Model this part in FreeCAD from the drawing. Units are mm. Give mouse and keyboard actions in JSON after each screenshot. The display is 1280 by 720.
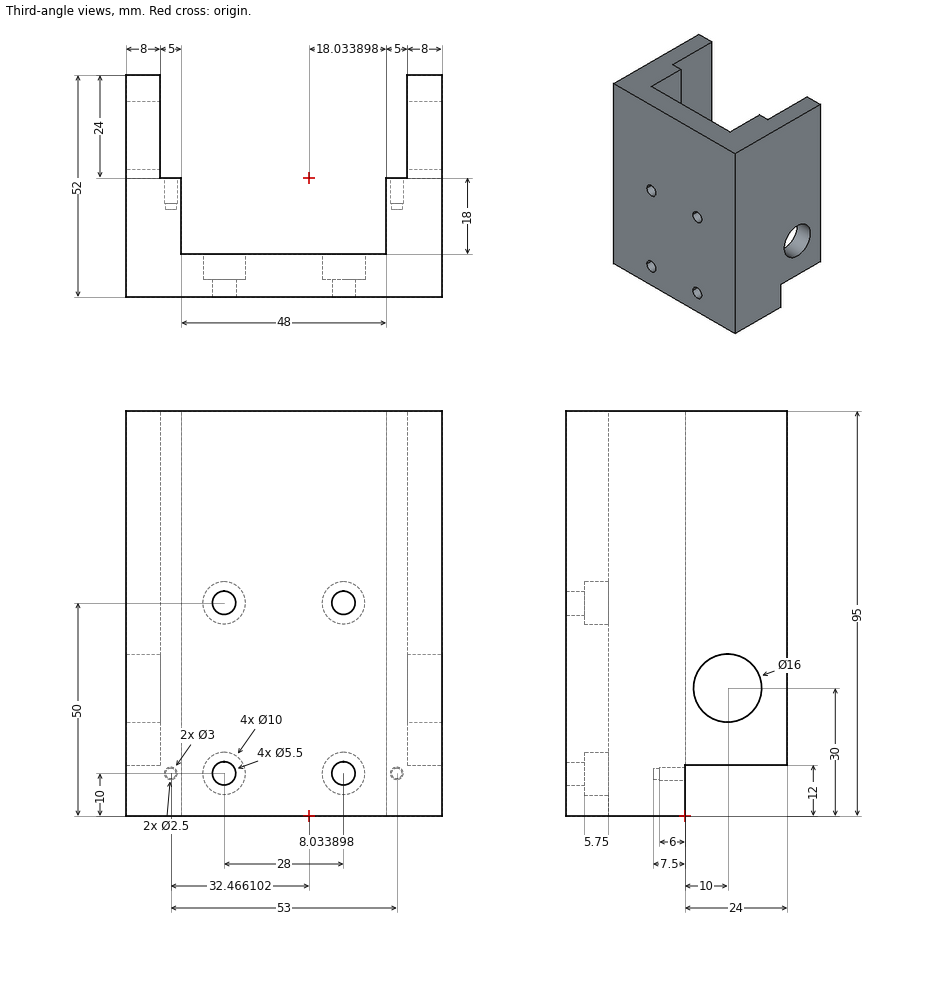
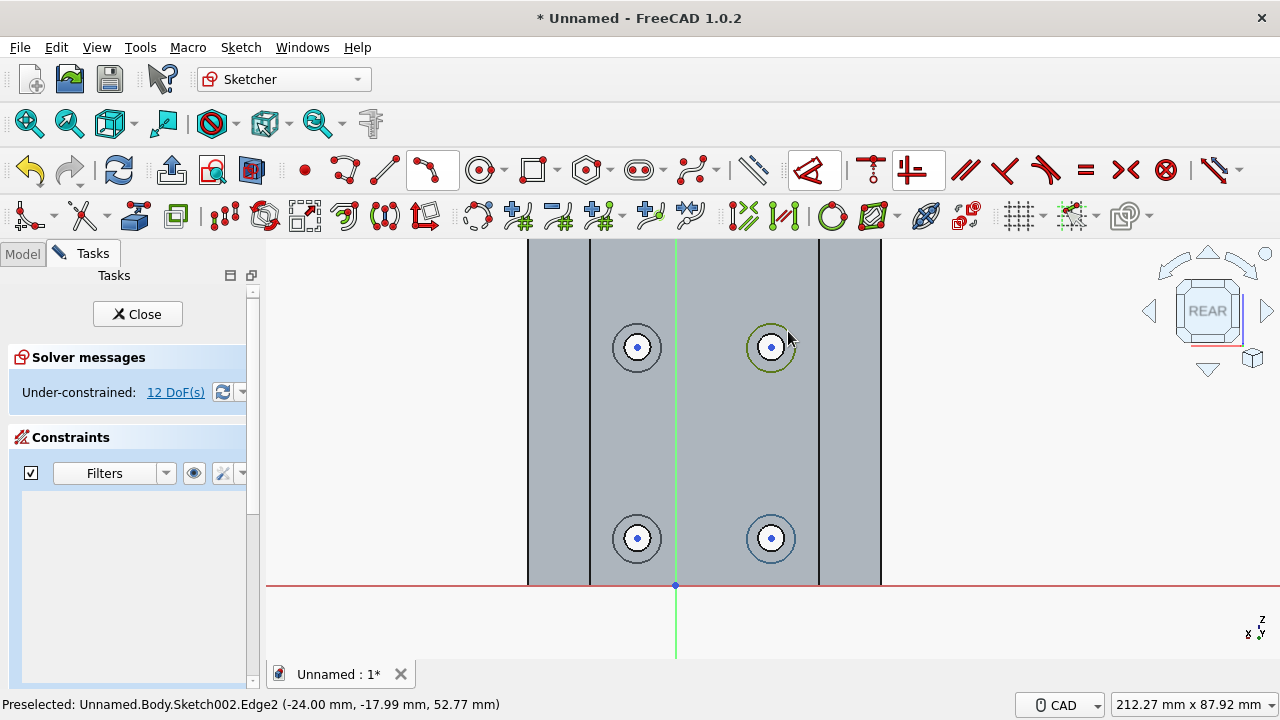
{"action": "left_click", "coordinate": [654, 522]}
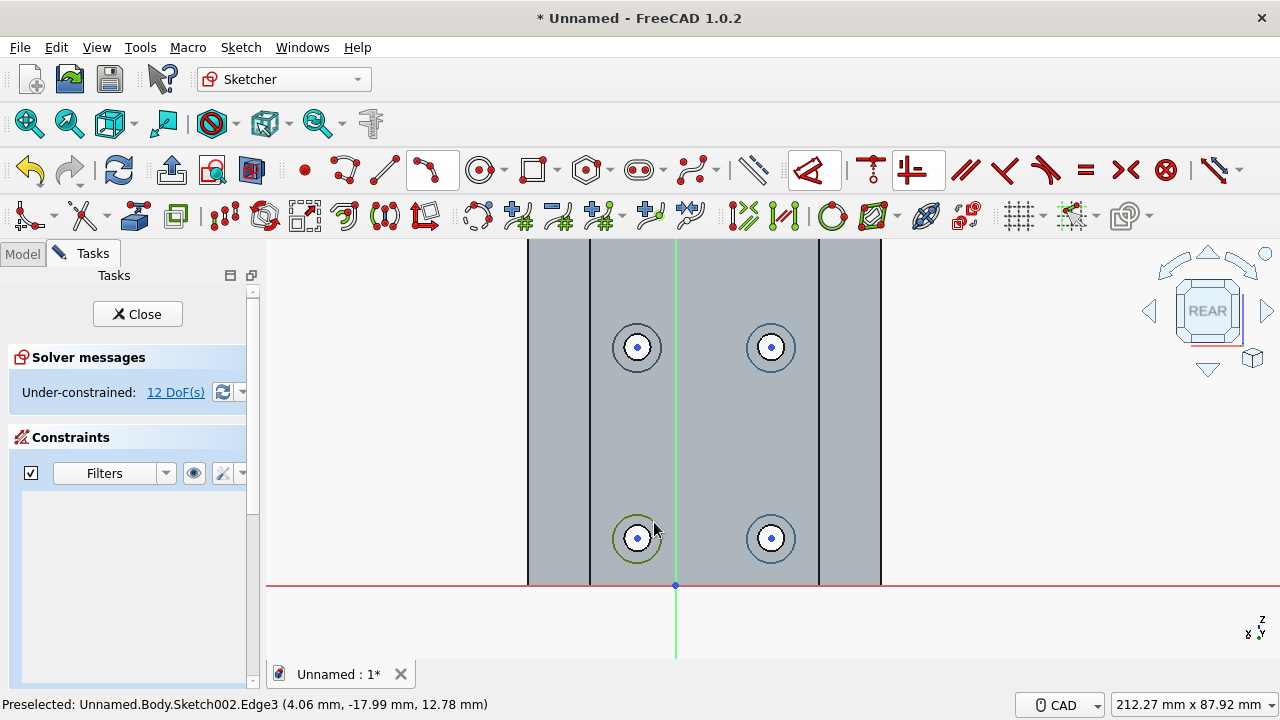
{"action": "left_click", "coordinate": [654, 331]}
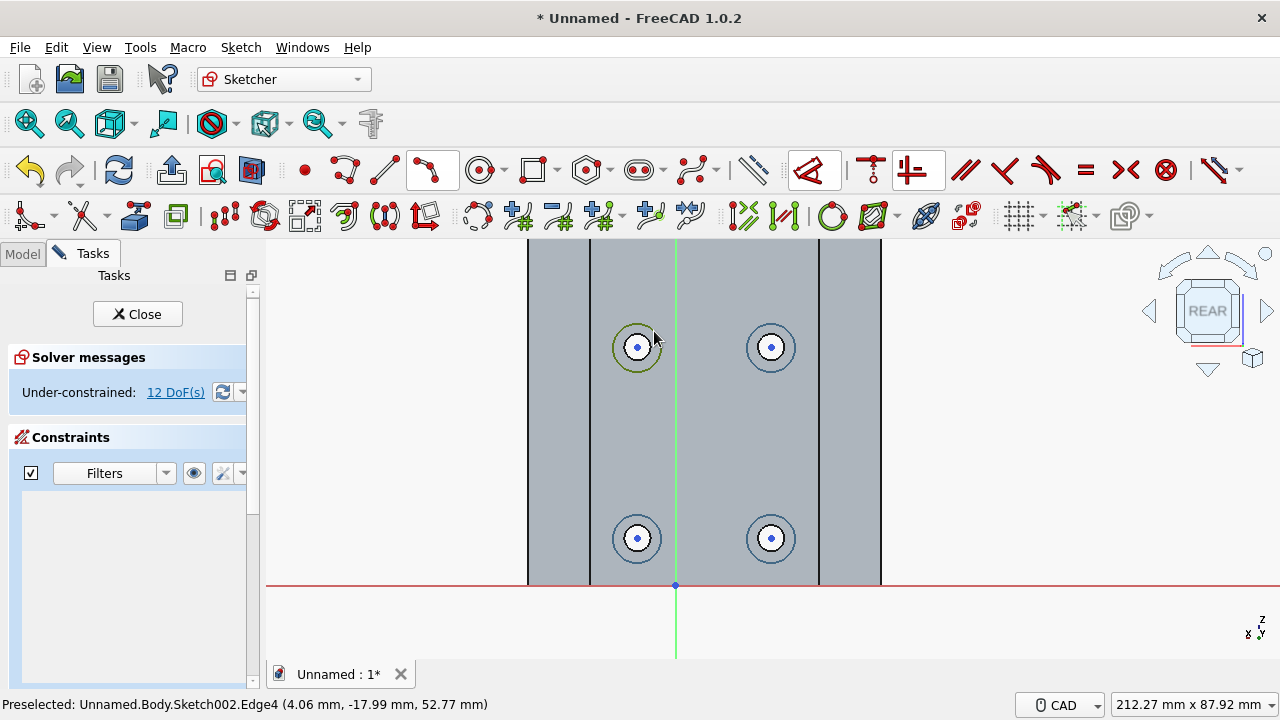
{"action": "key", "text": "e"}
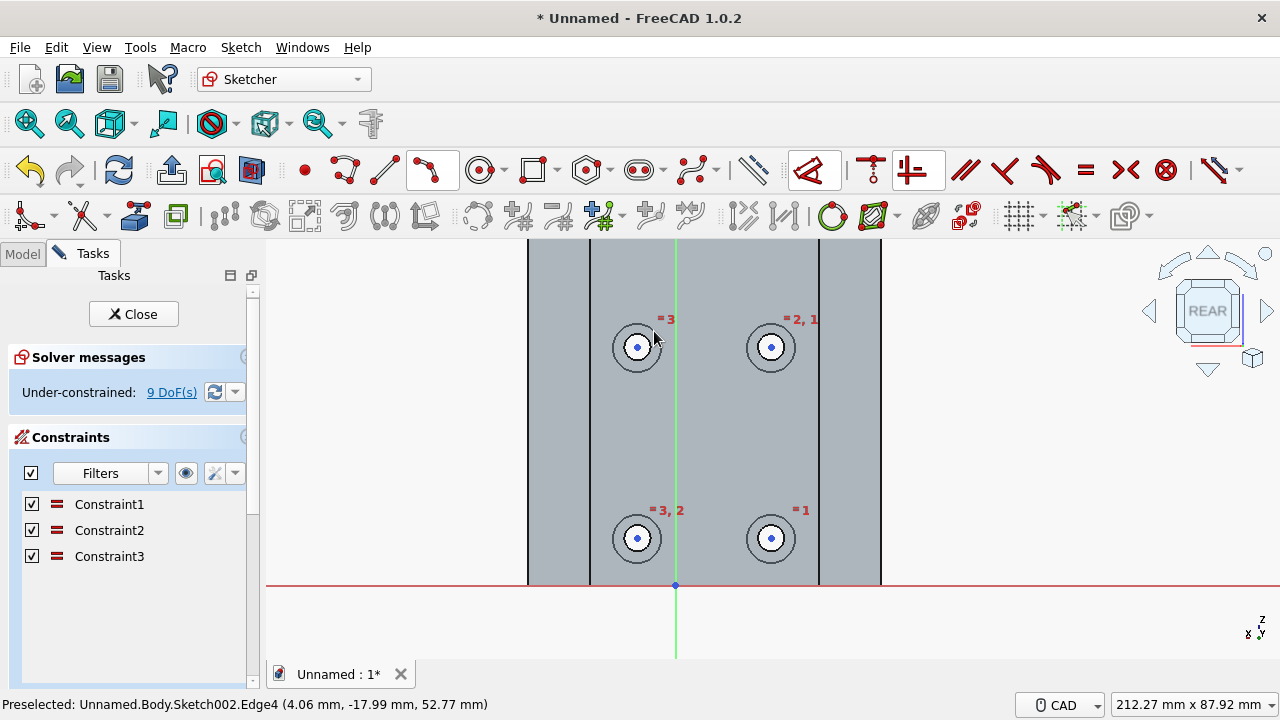
{"action": "left_click", "coordinate": [771, 539]}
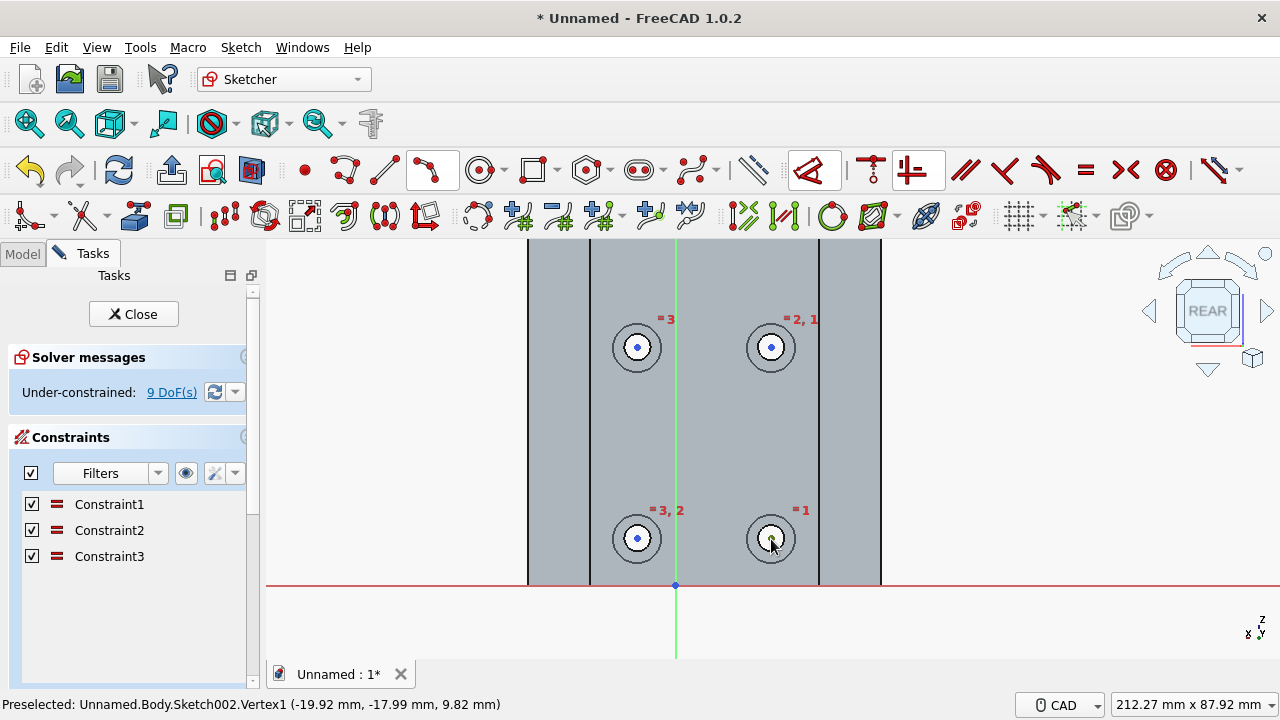
{"action": "left_click", "coordinate": [771, 348]}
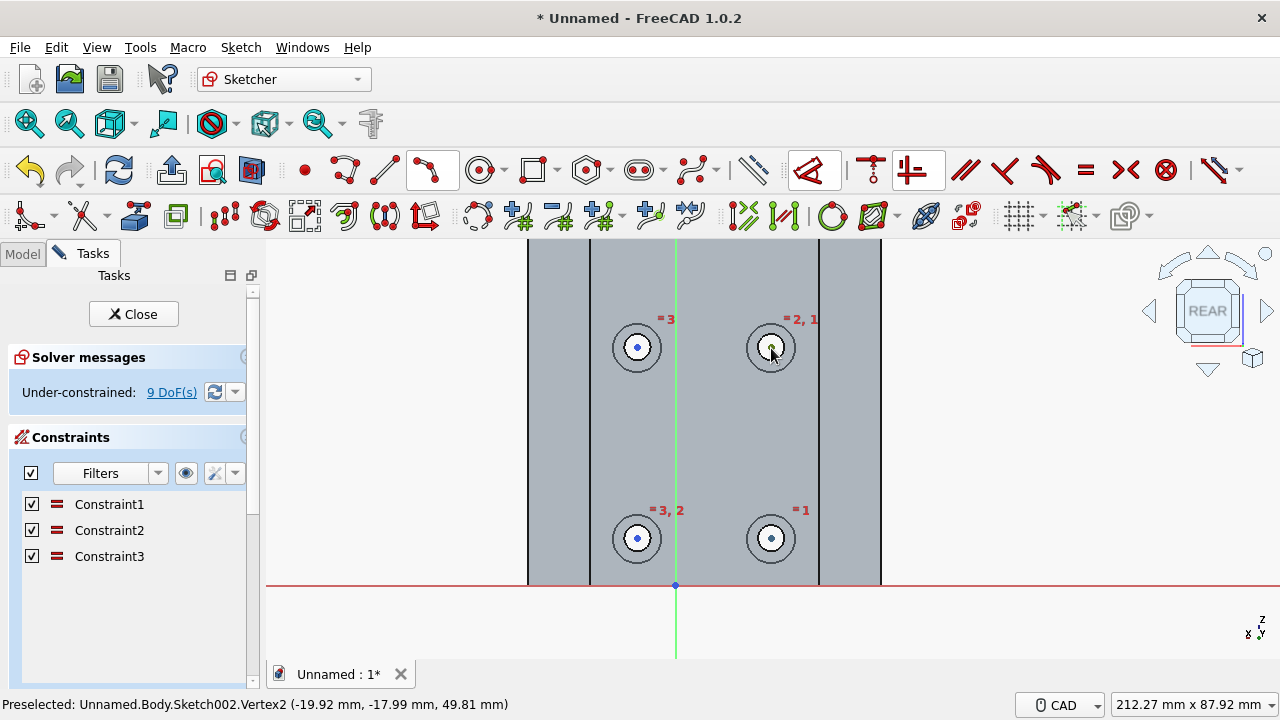
{"action": "key", "text": "v"}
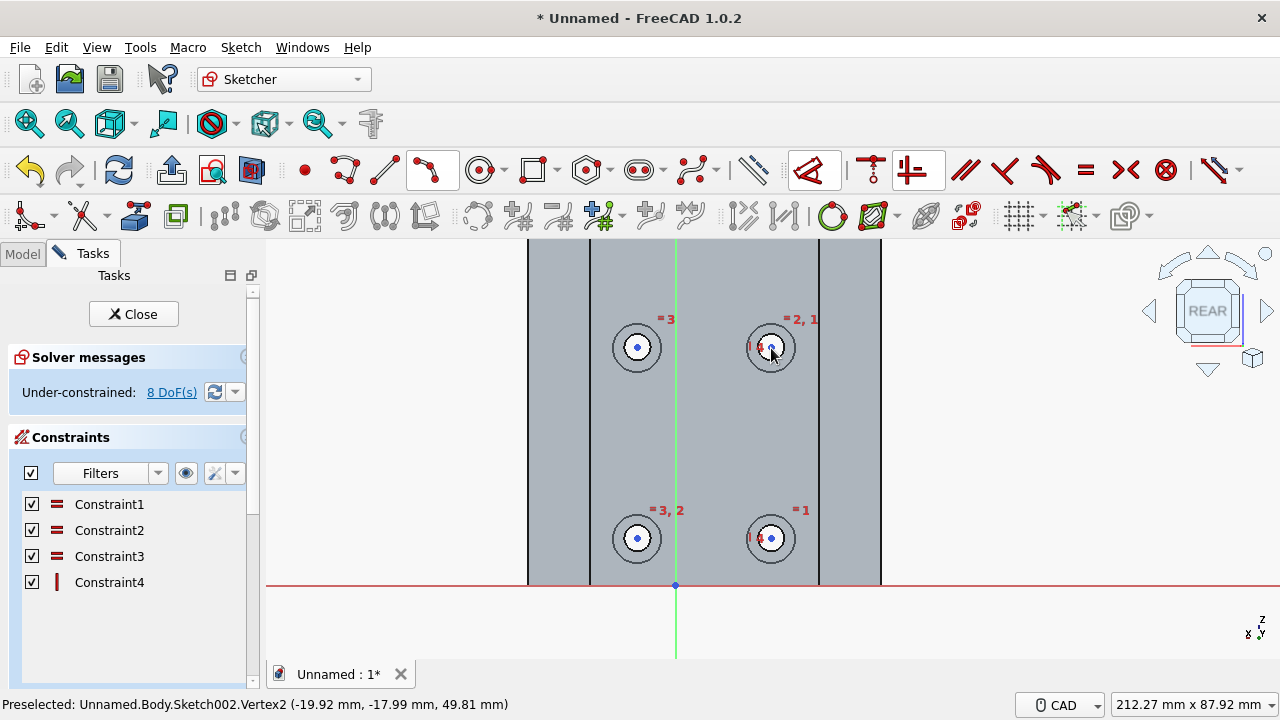
{"action": "left_click", "coordinate": [771, 539]}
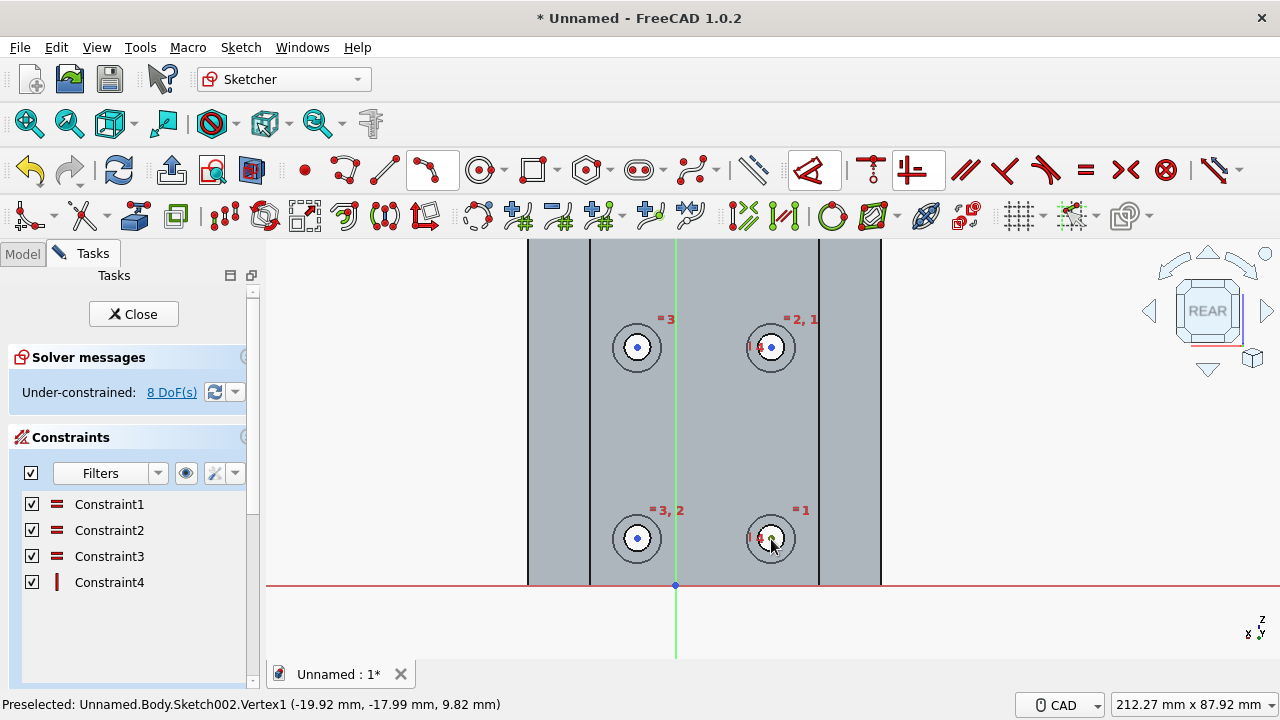
{"action": "left_click", "coordinate": [637, 539]}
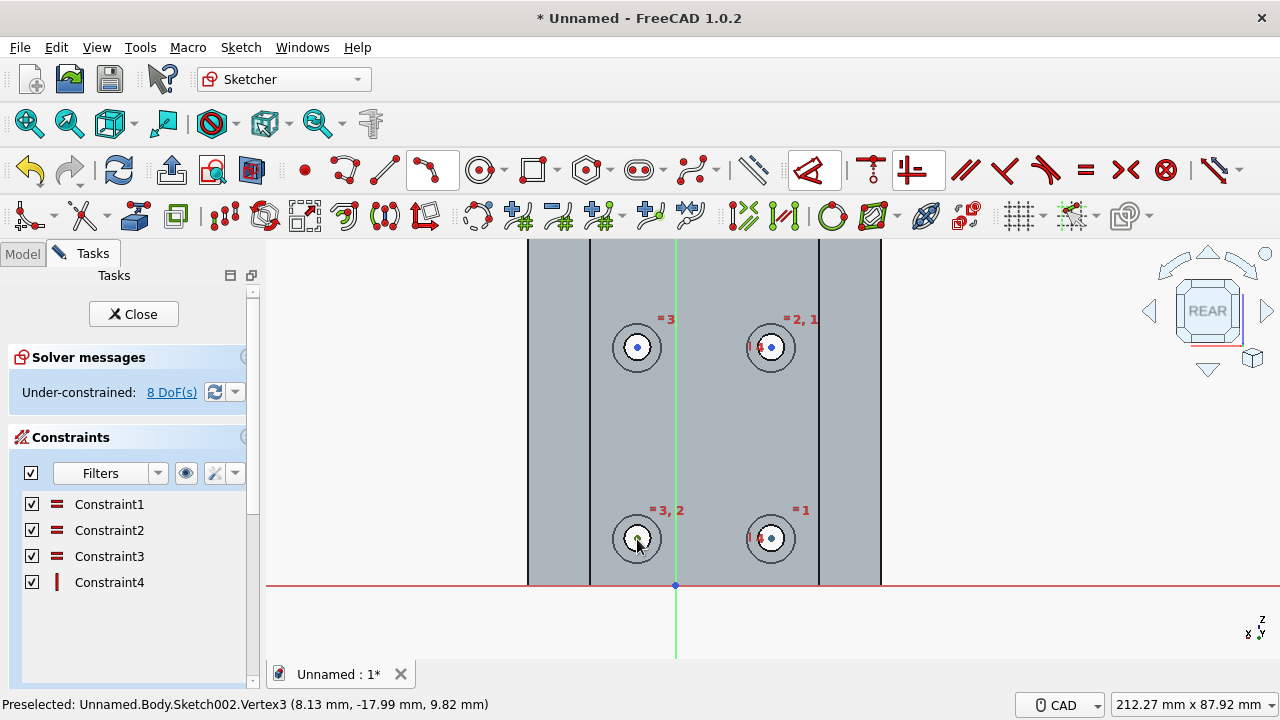
{"action": "left_click", "coordinate": [940, 170]}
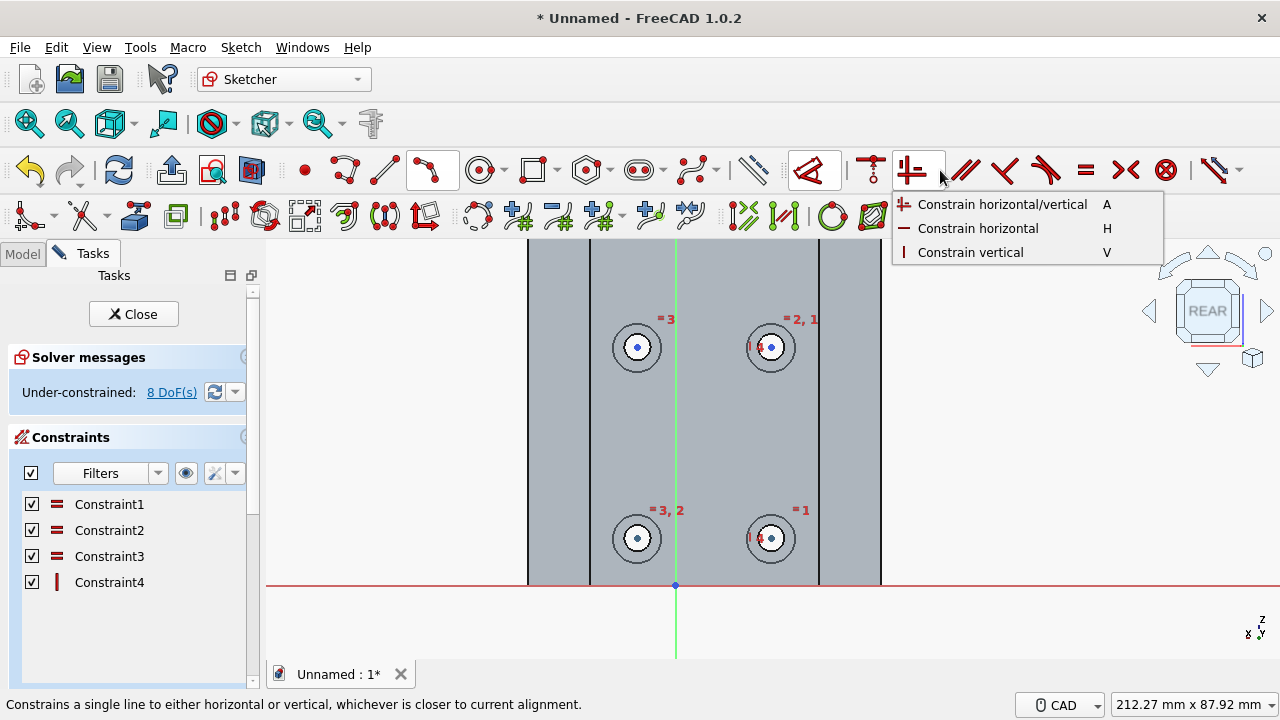
{"action": "left_click", "coordinate": [1028, 228]}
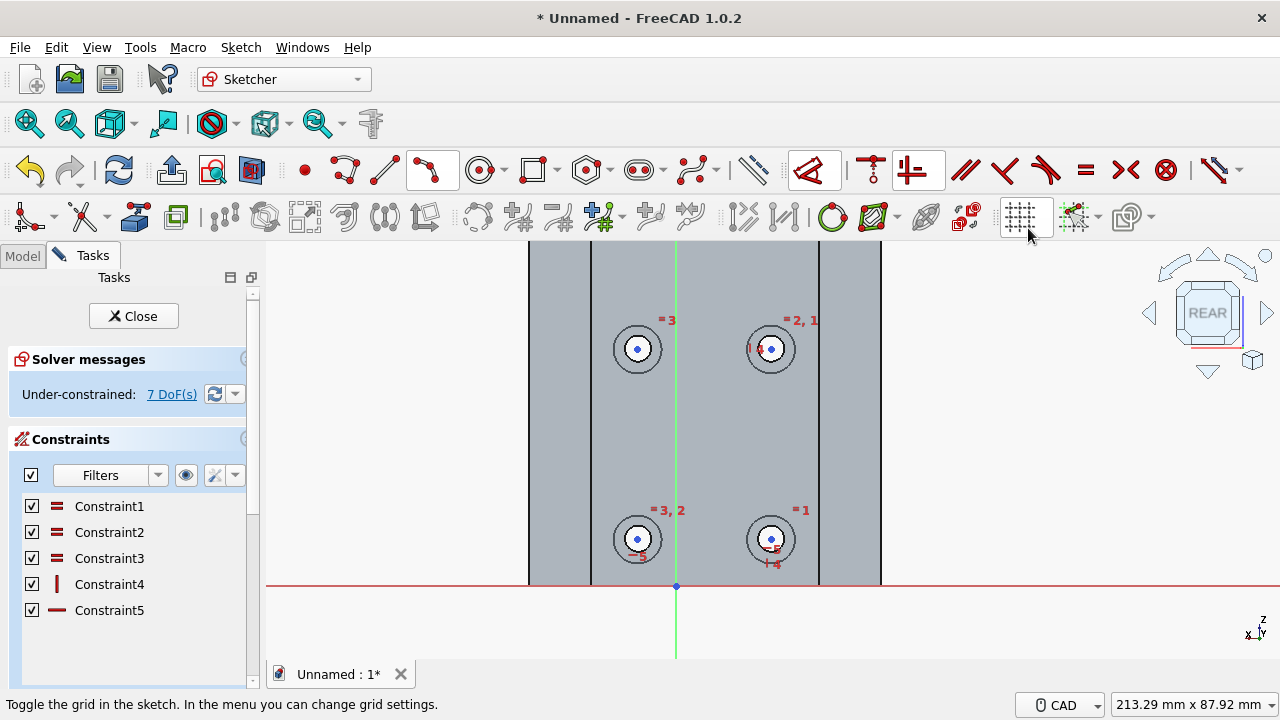
{"action": "left_click", "coordinate": [638, 540]}